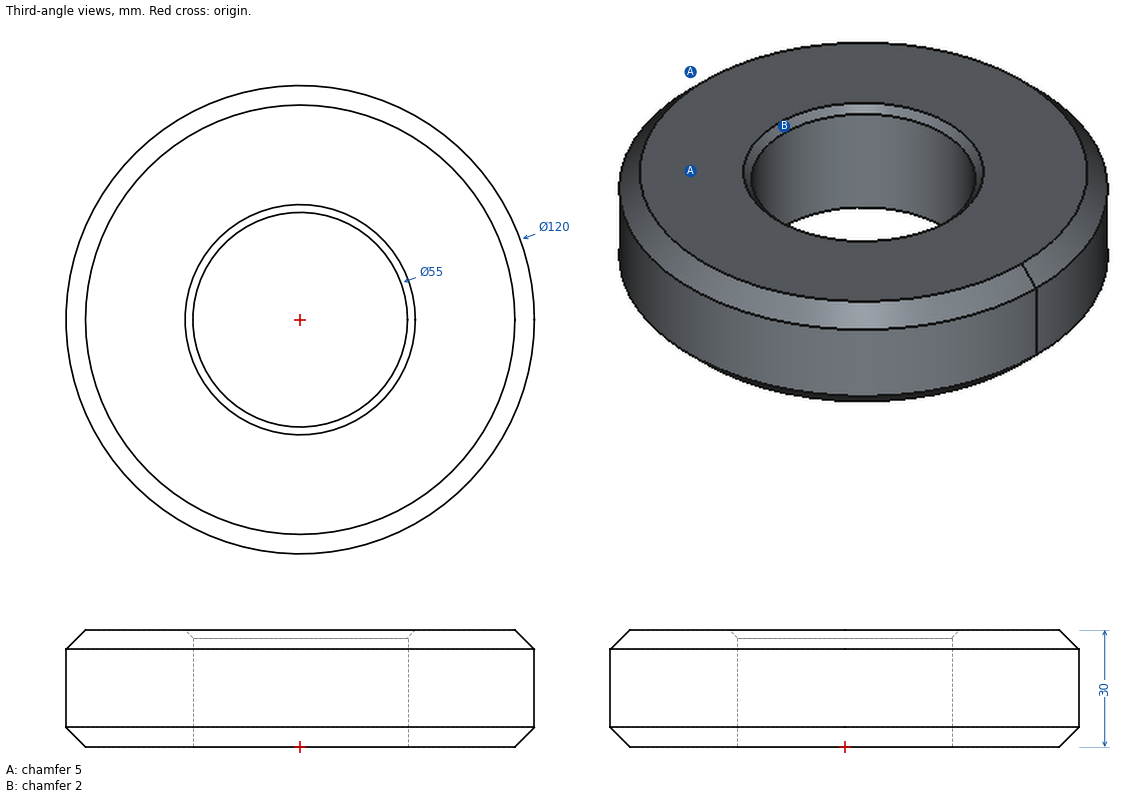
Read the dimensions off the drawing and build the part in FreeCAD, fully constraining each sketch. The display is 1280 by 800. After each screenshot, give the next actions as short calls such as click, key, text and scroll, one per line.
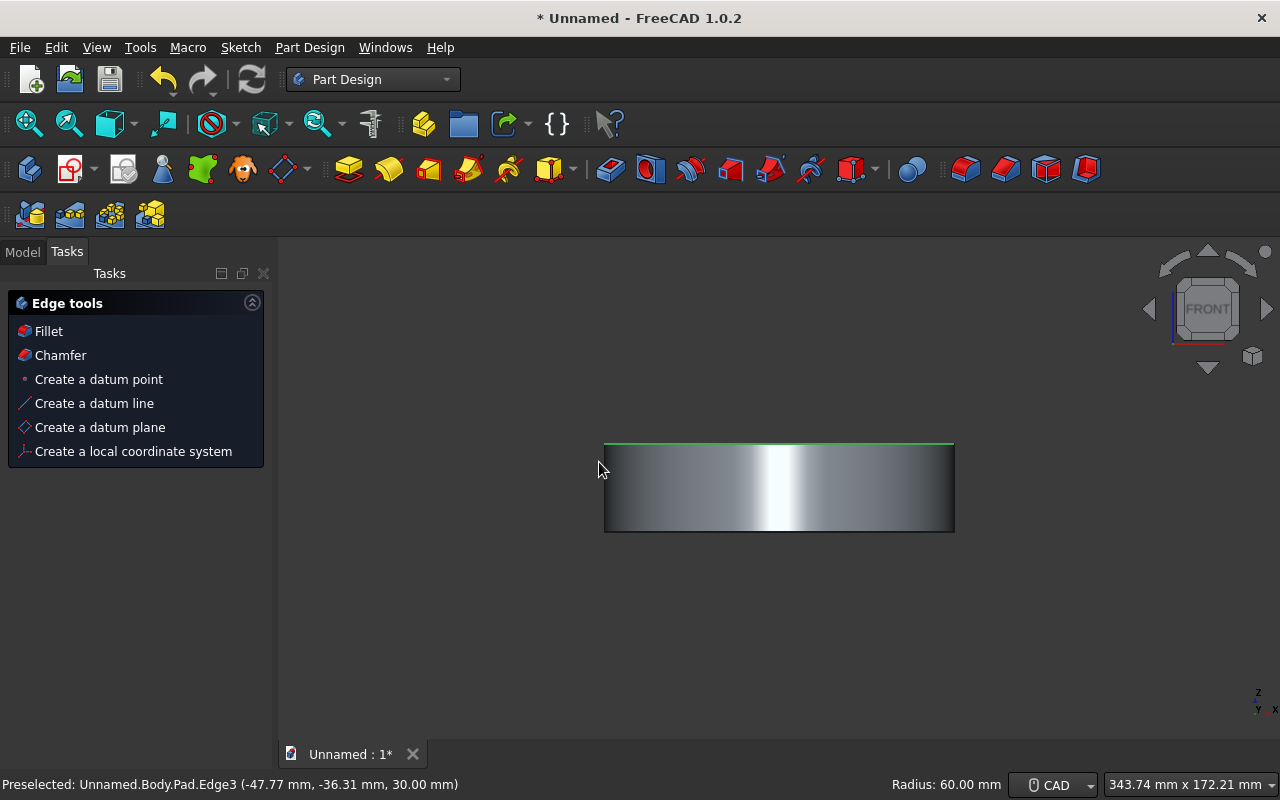
click(638, 531, ctrl)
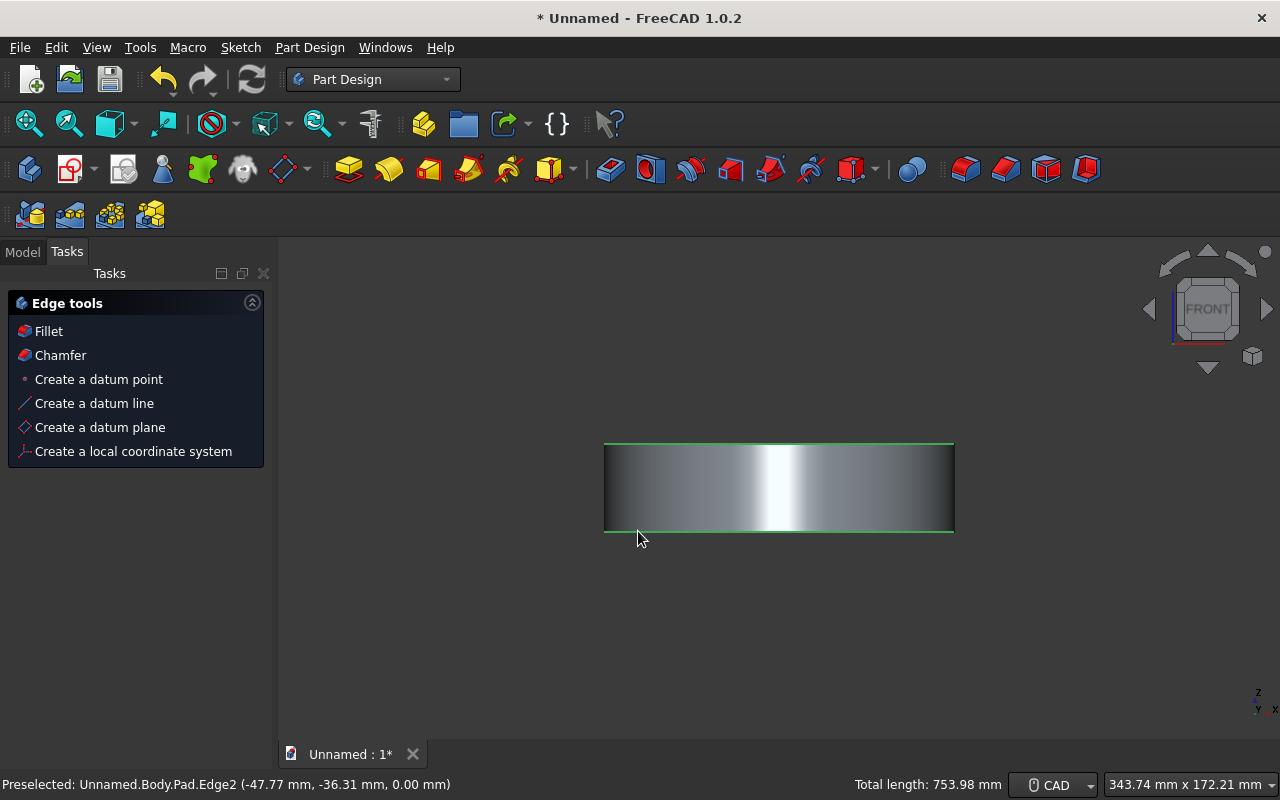
click(1006, 170)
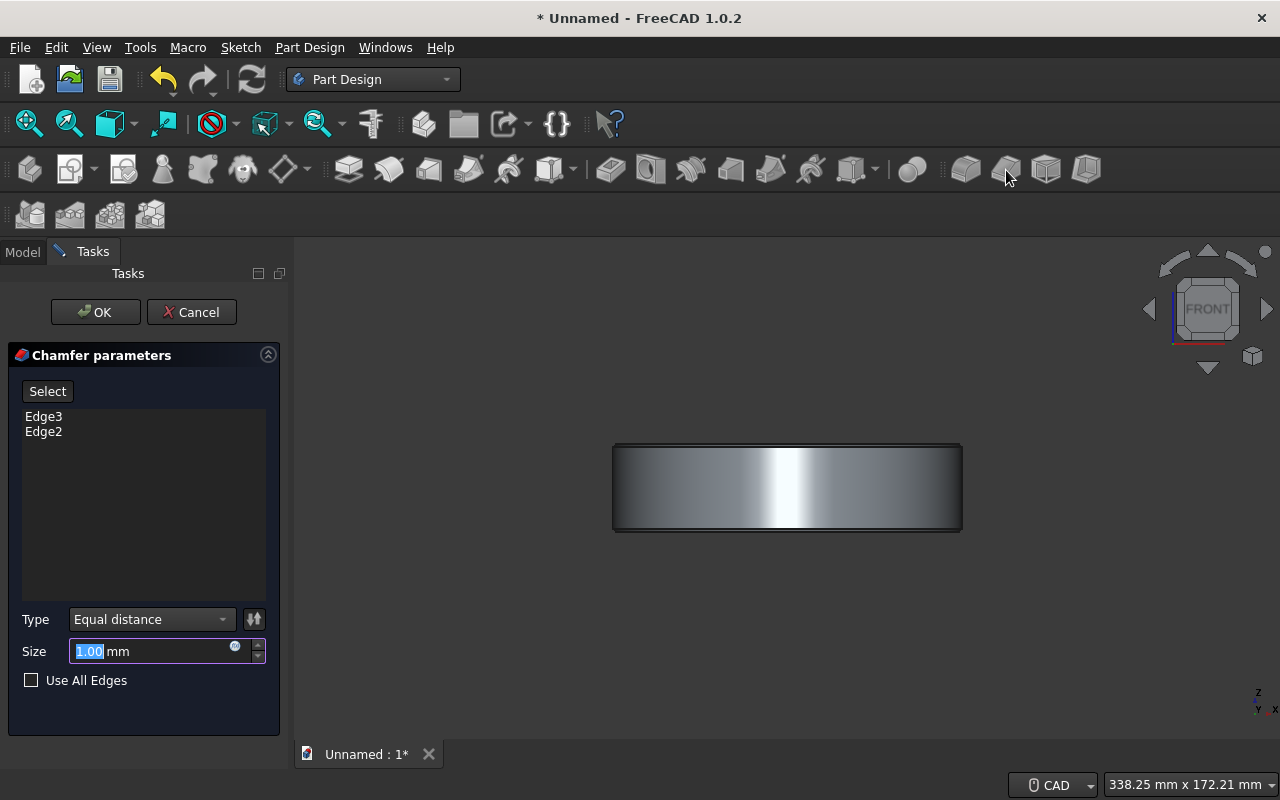
text(5)
key(Tab)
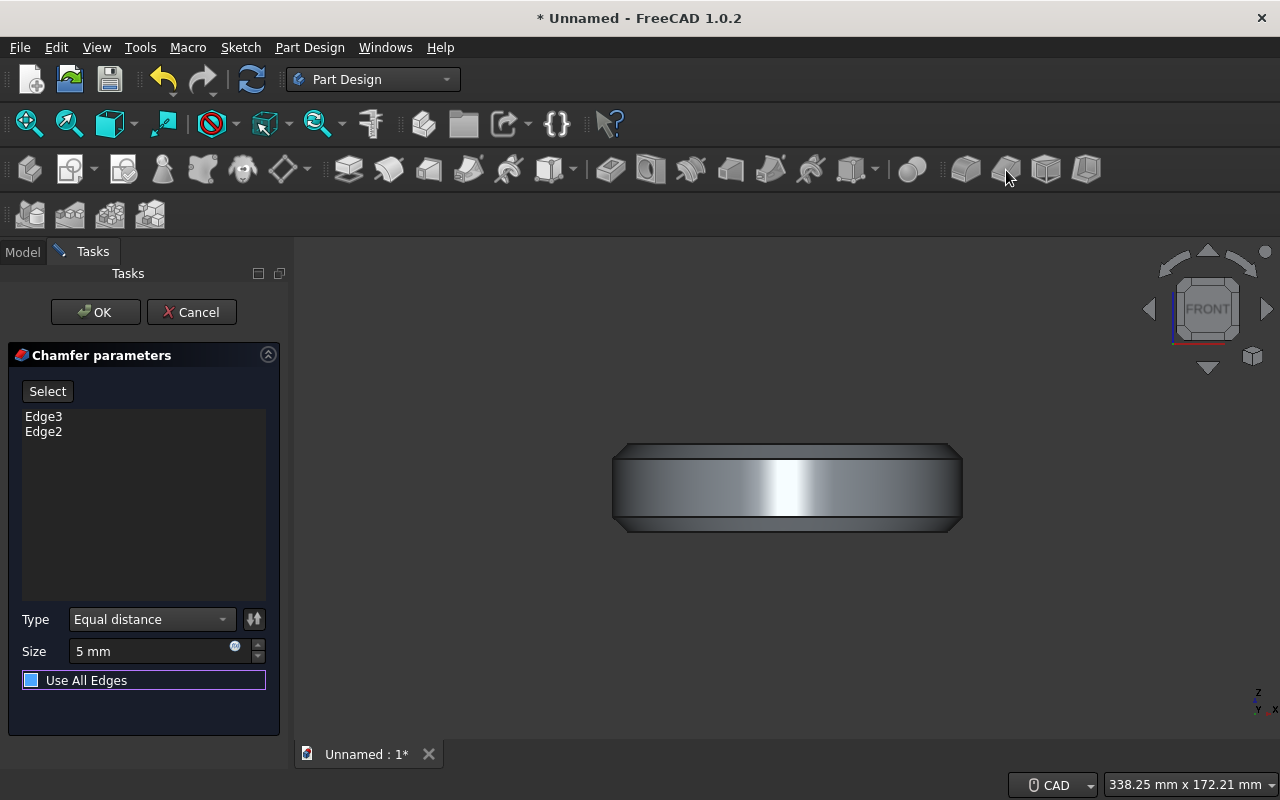
click(96, 312)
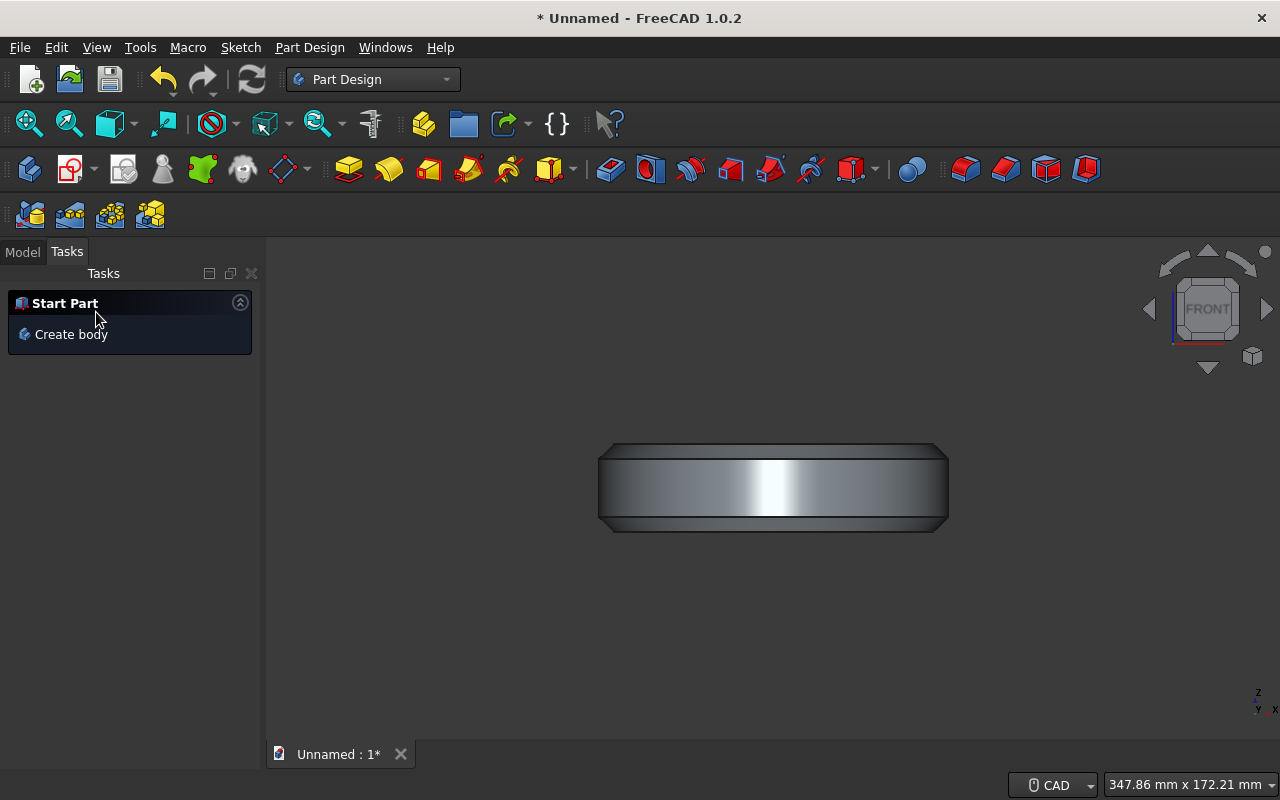
click(30, 124)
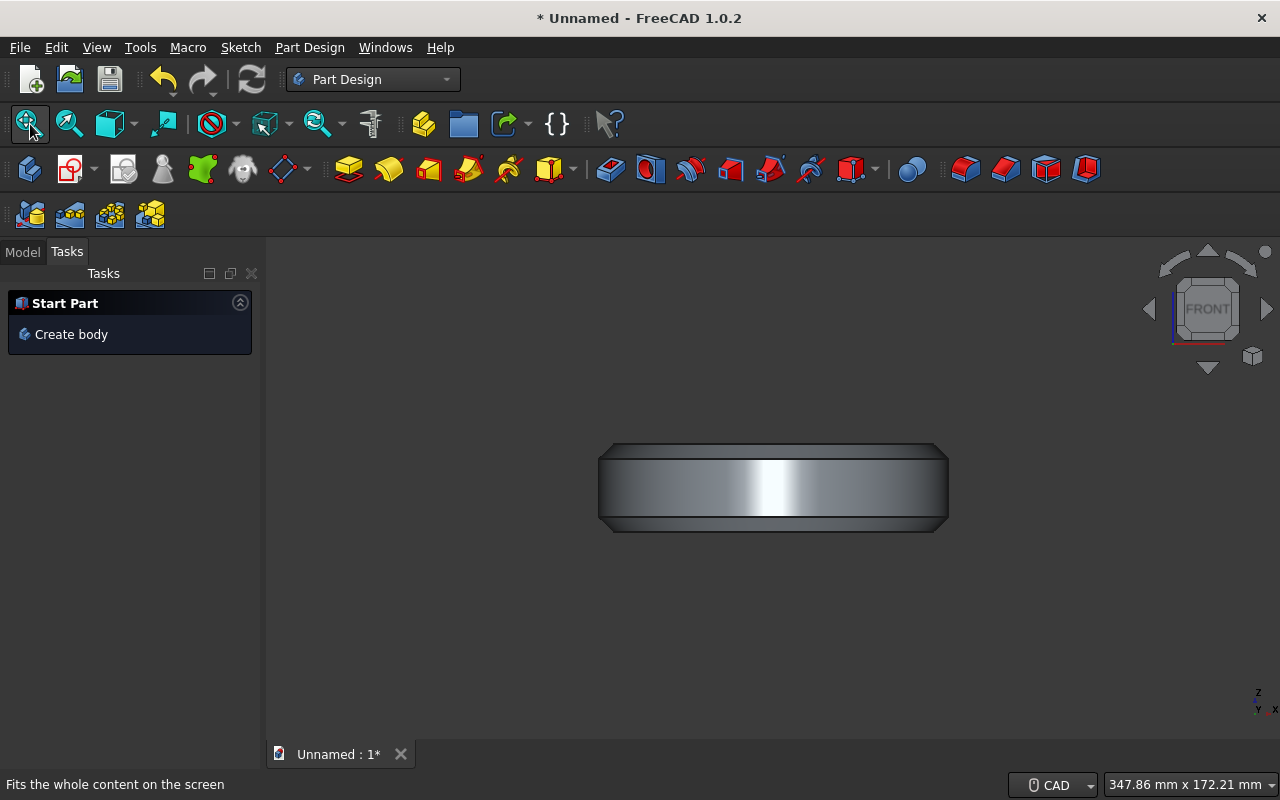
key(0)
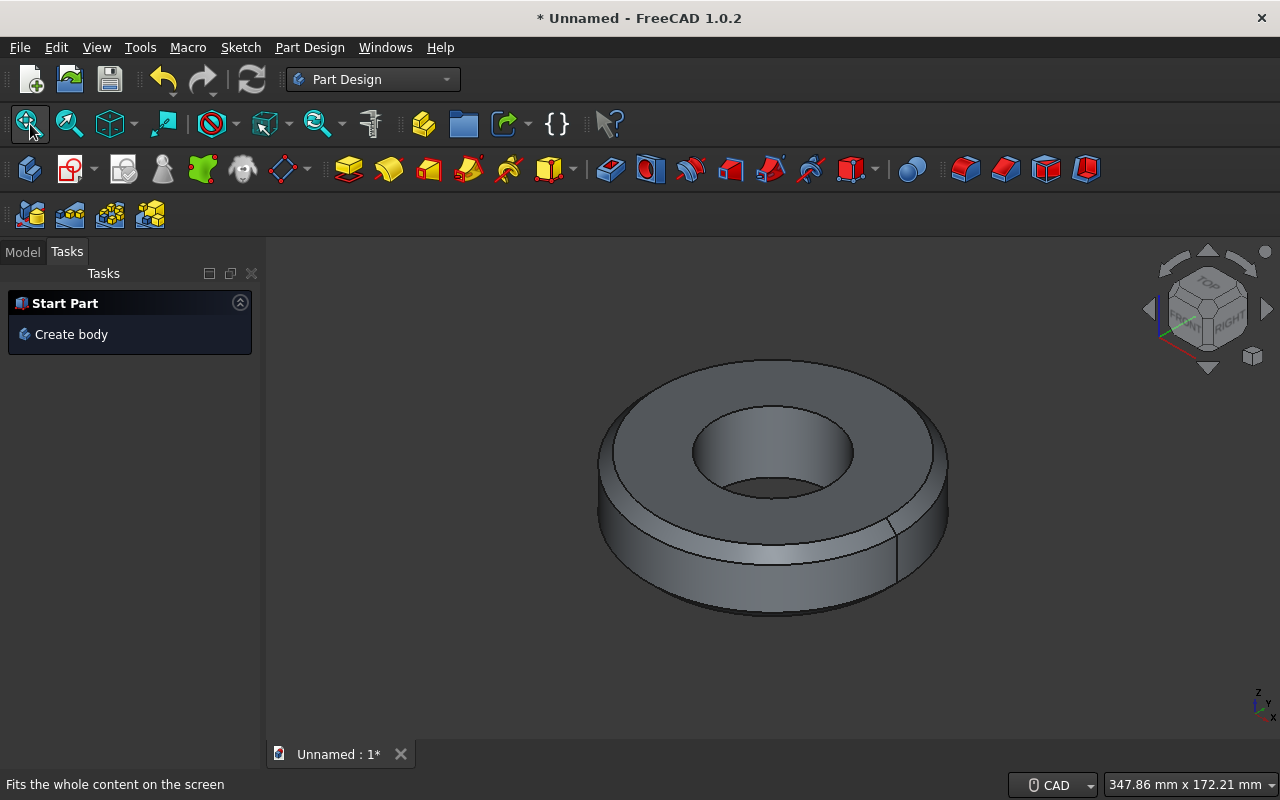
click(716, 419)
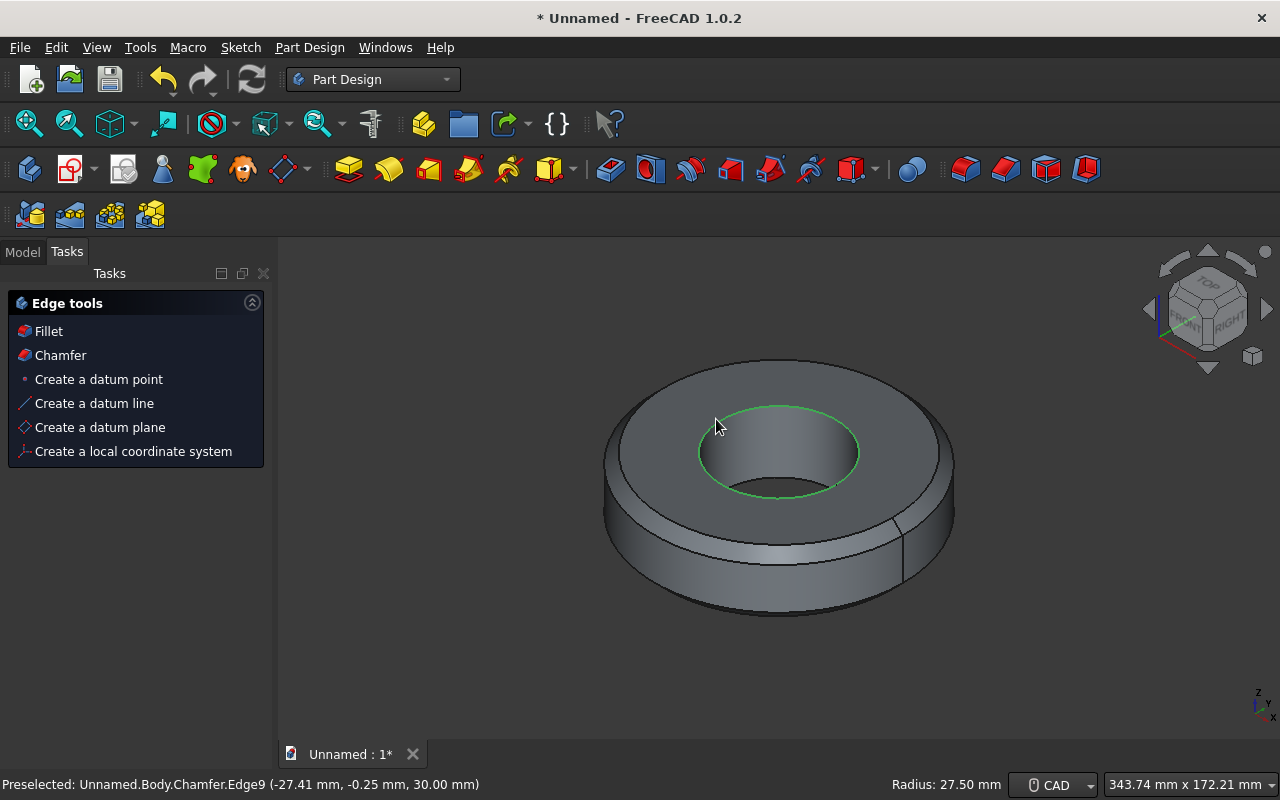
click(1006, 170)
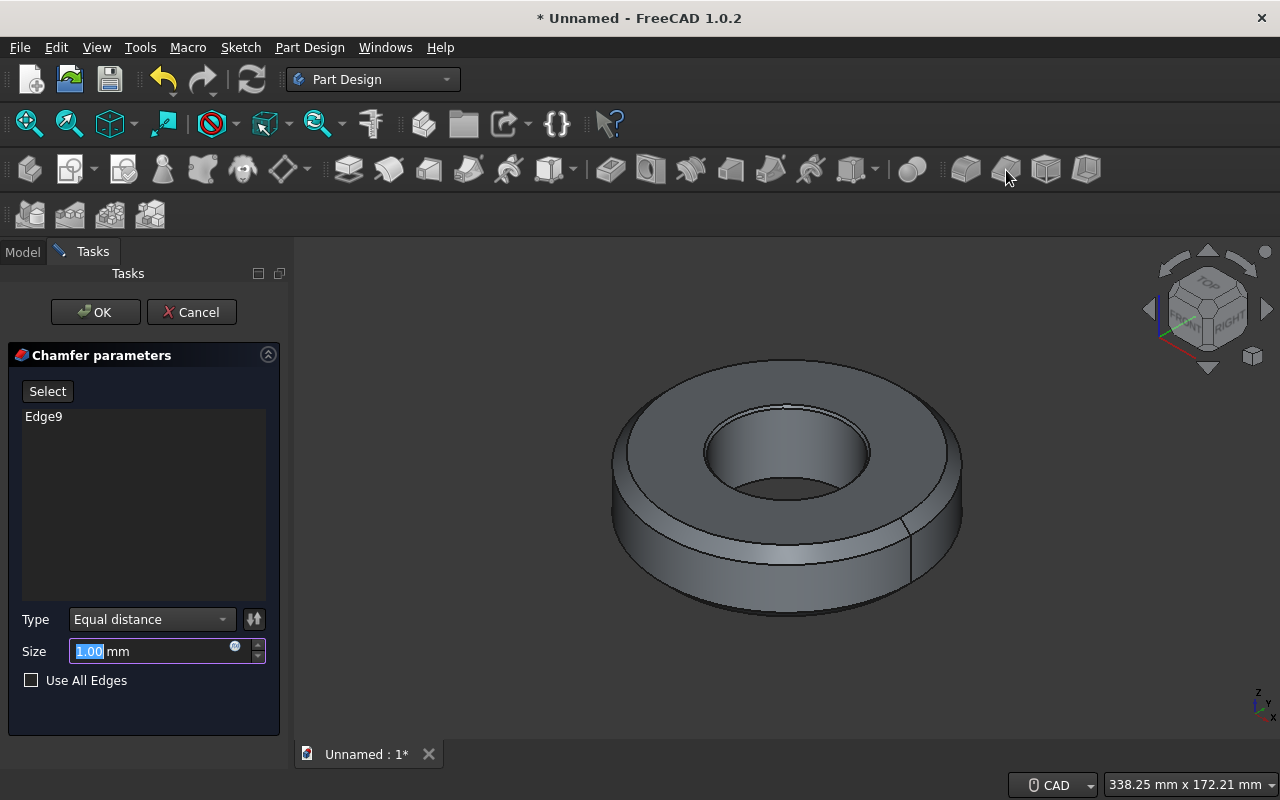
text(2)
key(Tab)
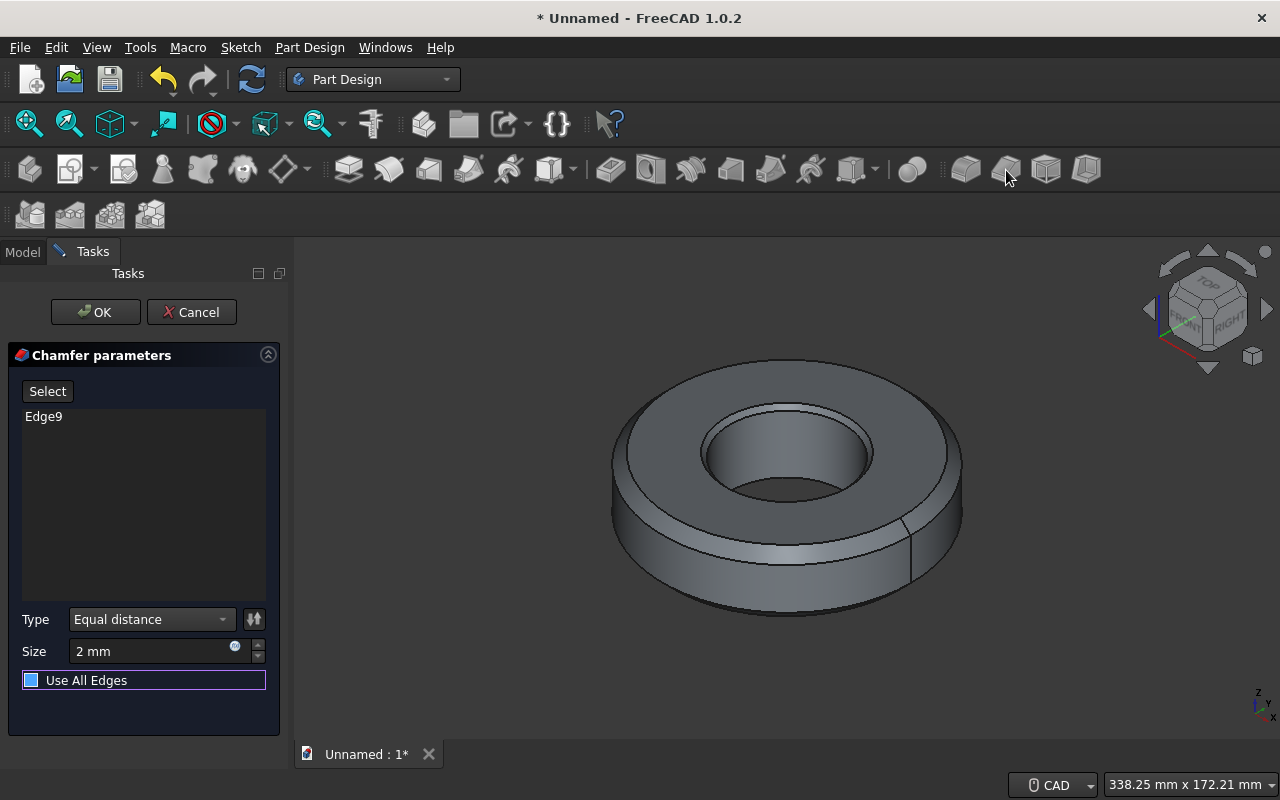
click(96, 312)